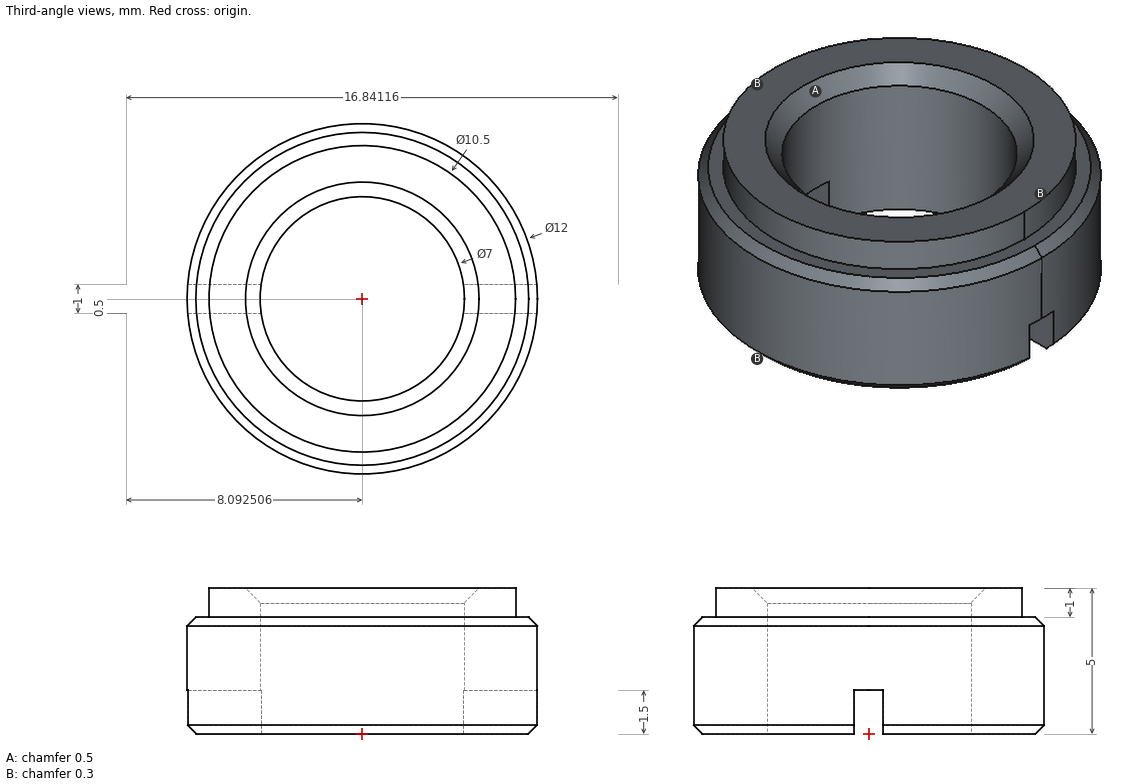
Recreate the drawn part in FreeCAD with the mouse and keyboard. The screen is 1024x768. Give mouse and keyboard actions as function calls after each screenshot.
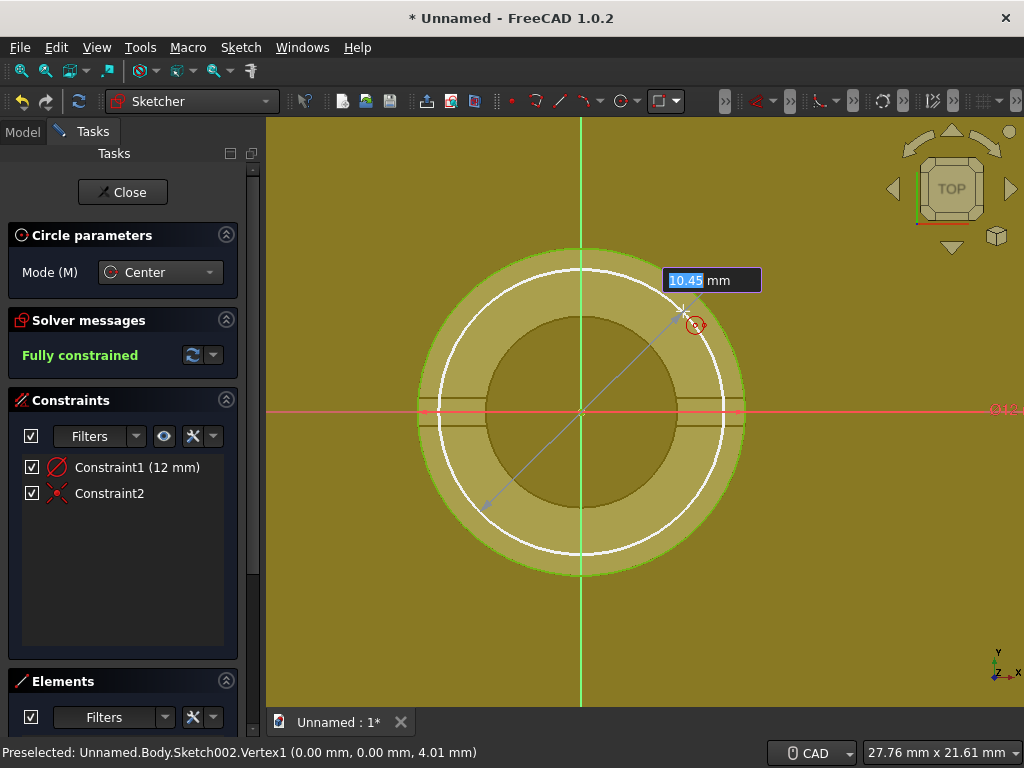
text(10.5)
key(Return)
key(Escape)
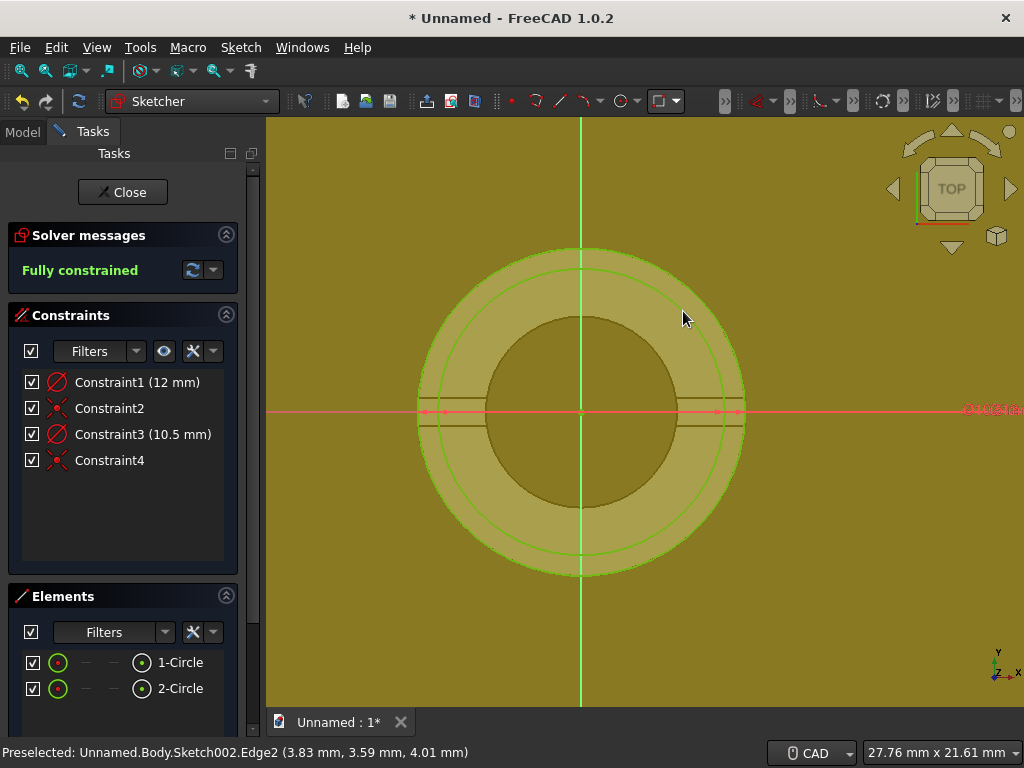
click(123, 192)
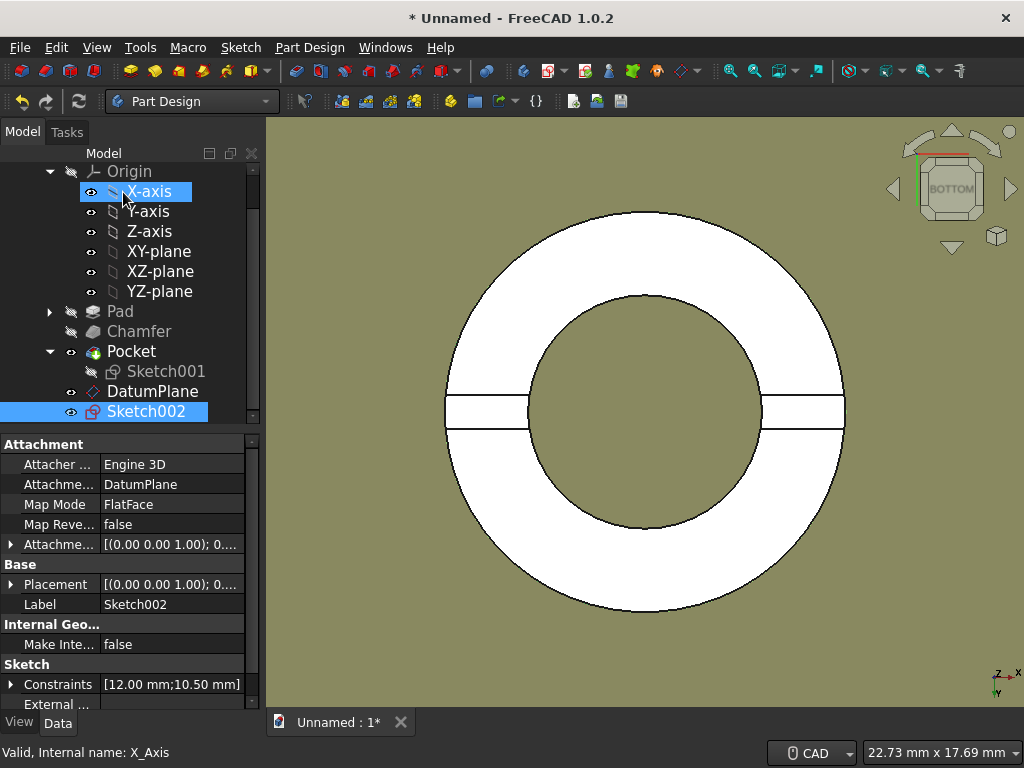
click(298, 72)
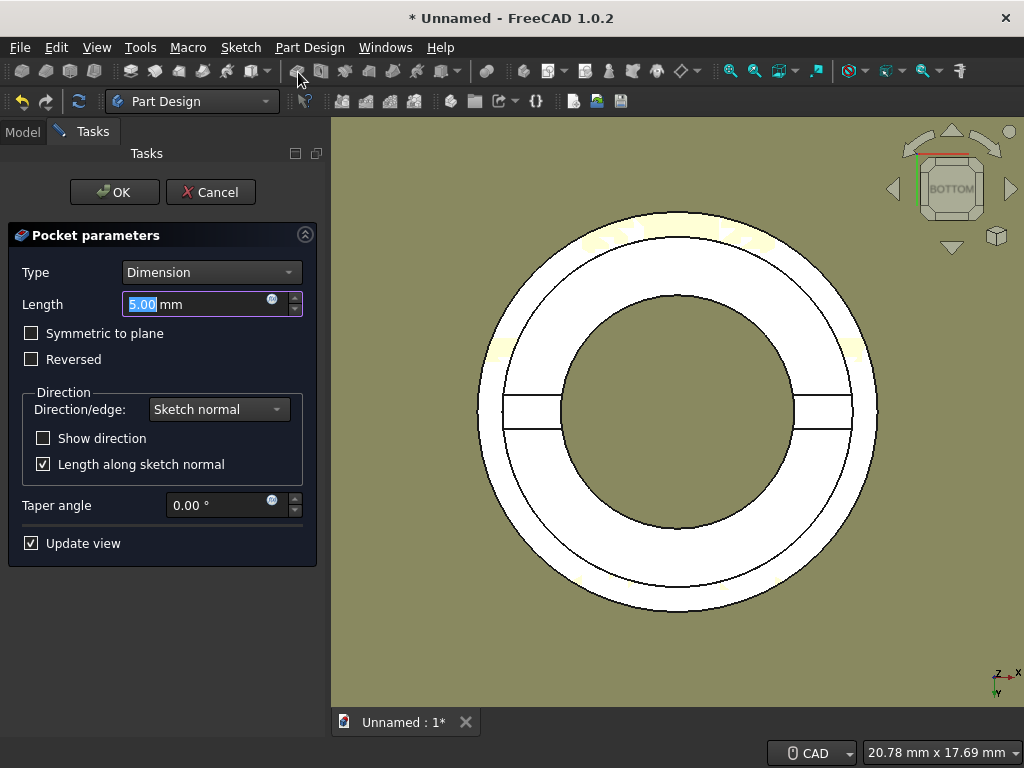
text(1)
key(Tab)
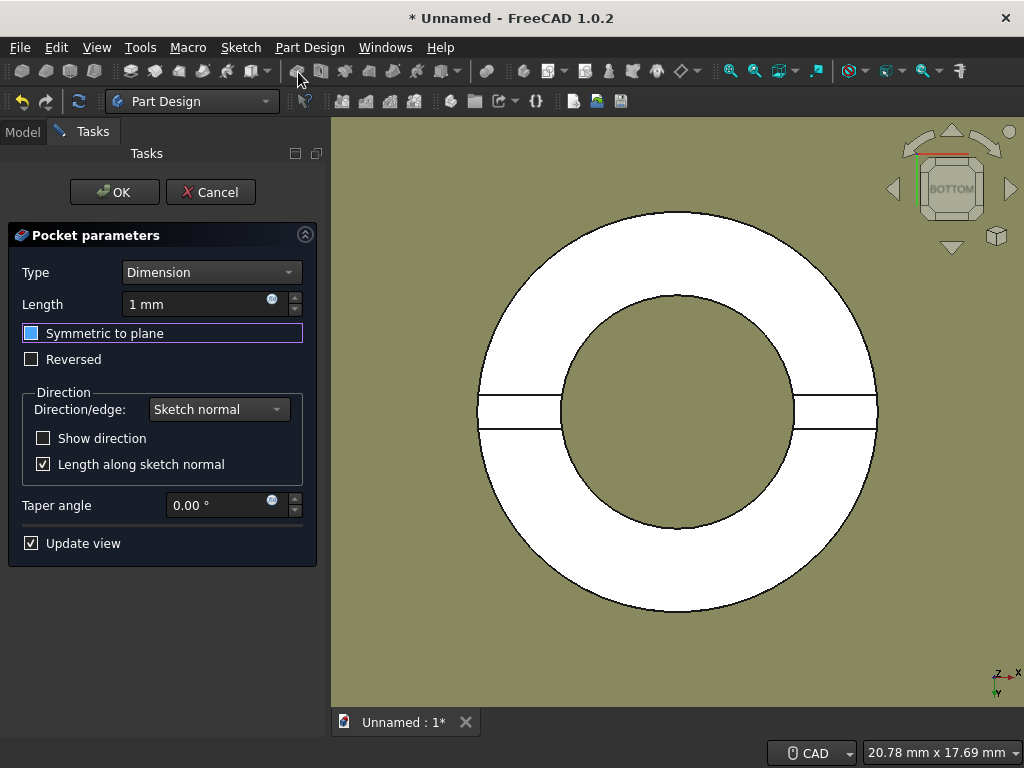
click(30, 359)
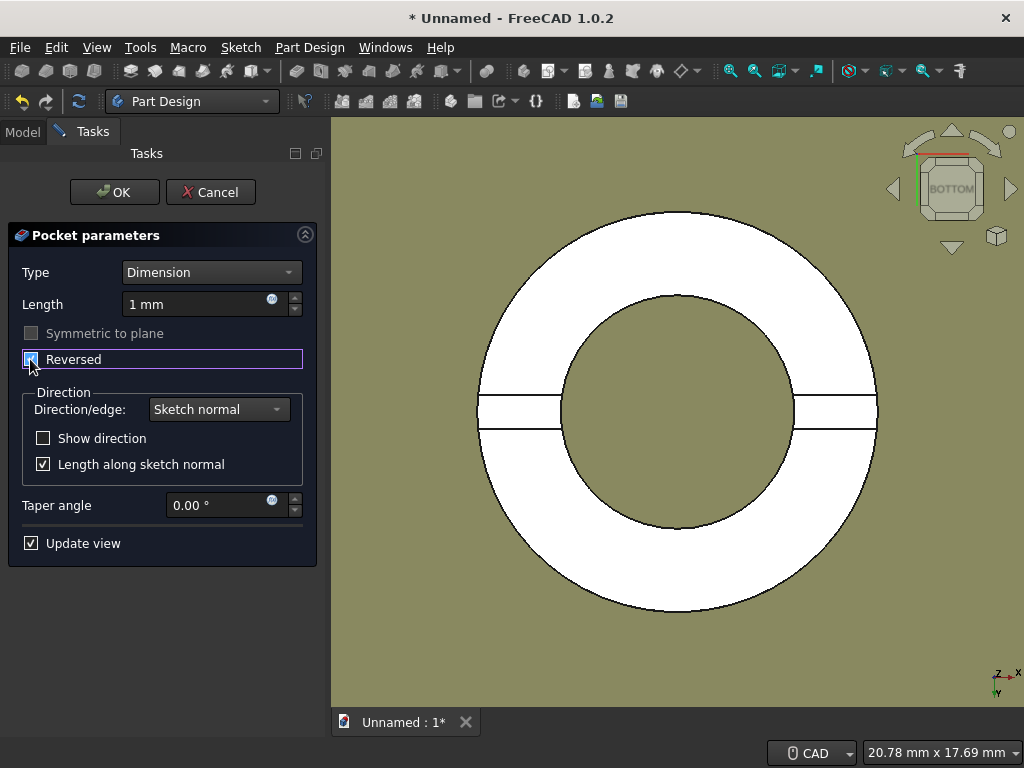
click(115, 192)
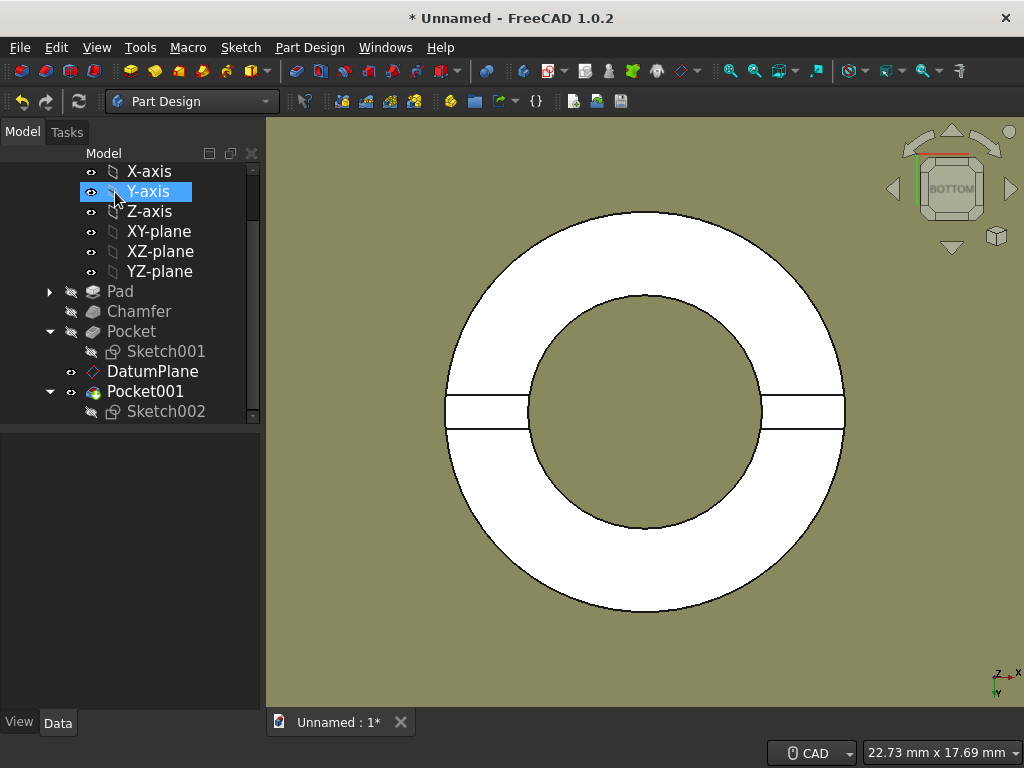
click(116, 372)
key(space)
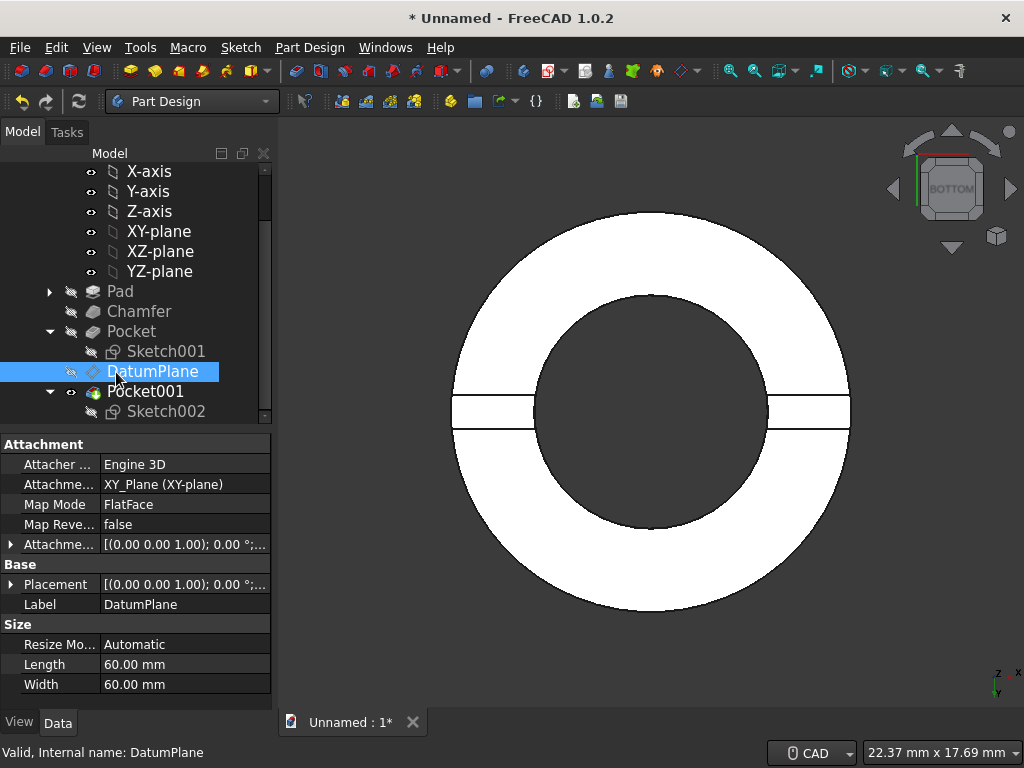
click(539, 245)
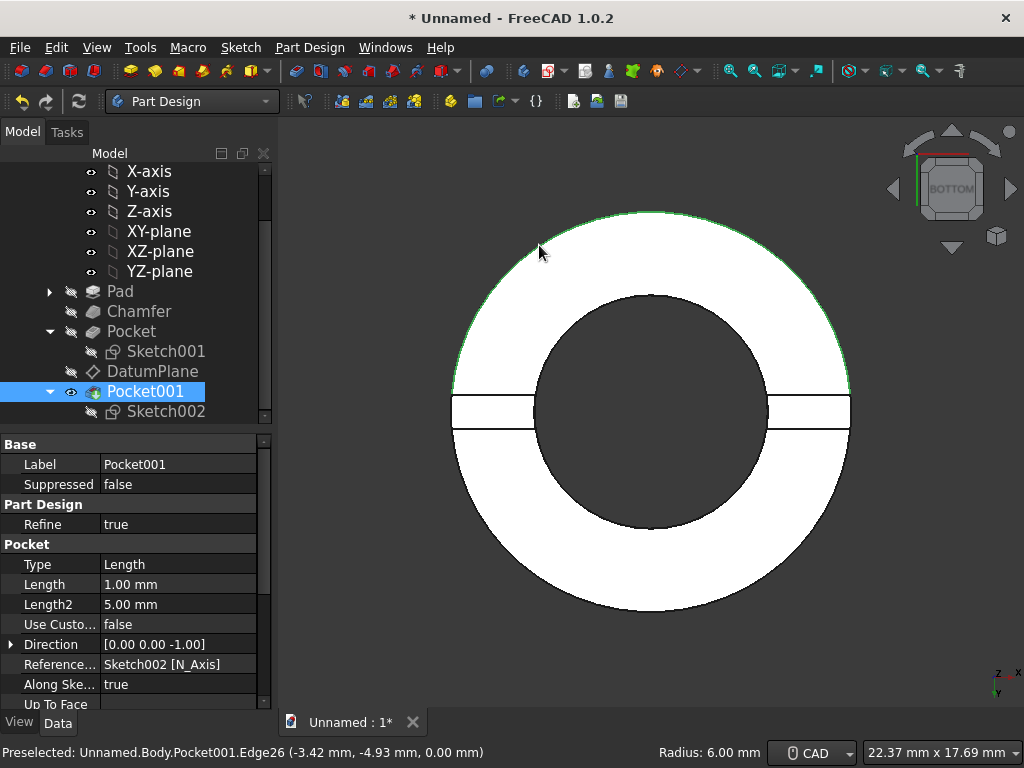
click(651, 611, ctrl)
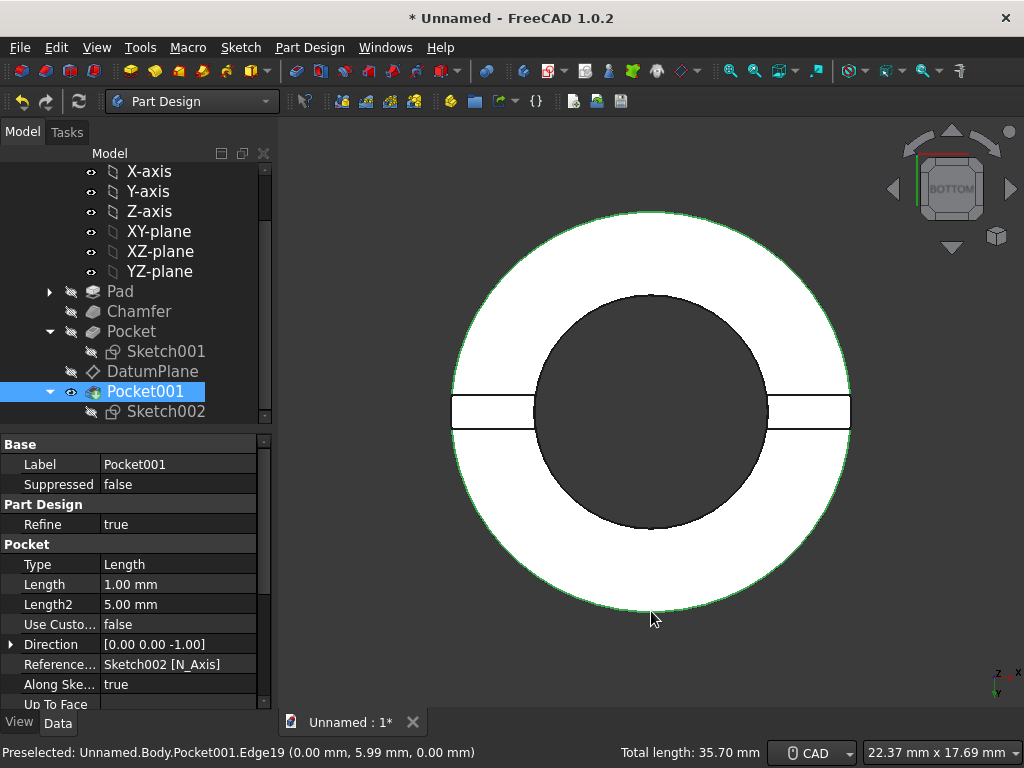
key(0)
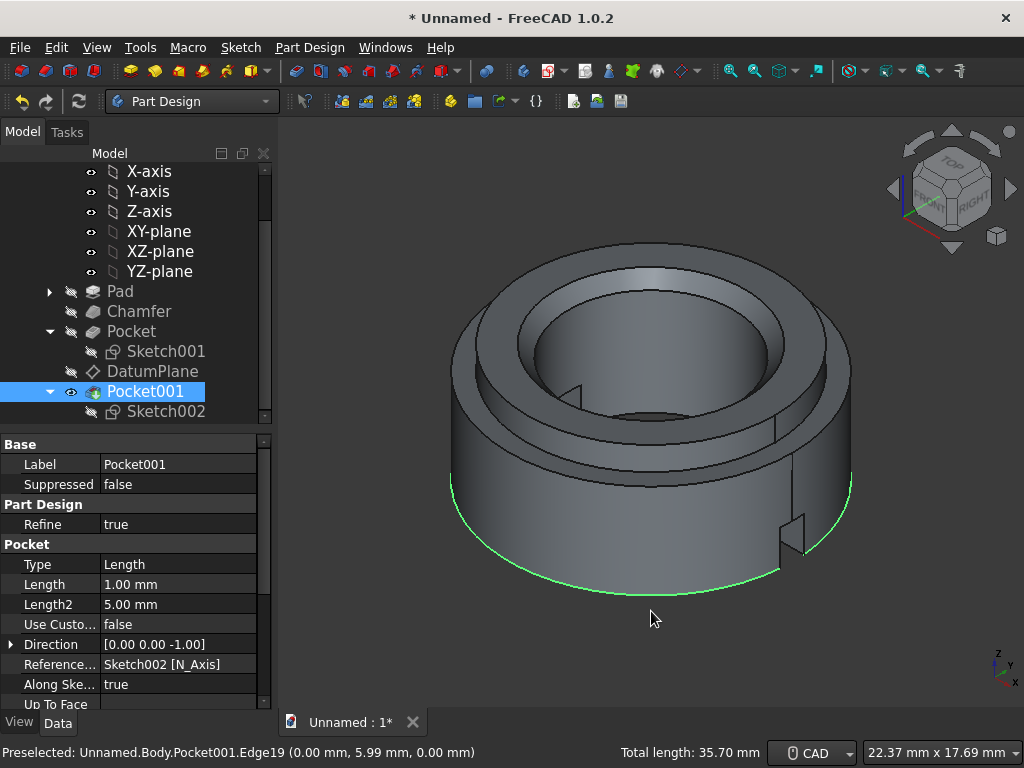
click(473, 423, ctrl)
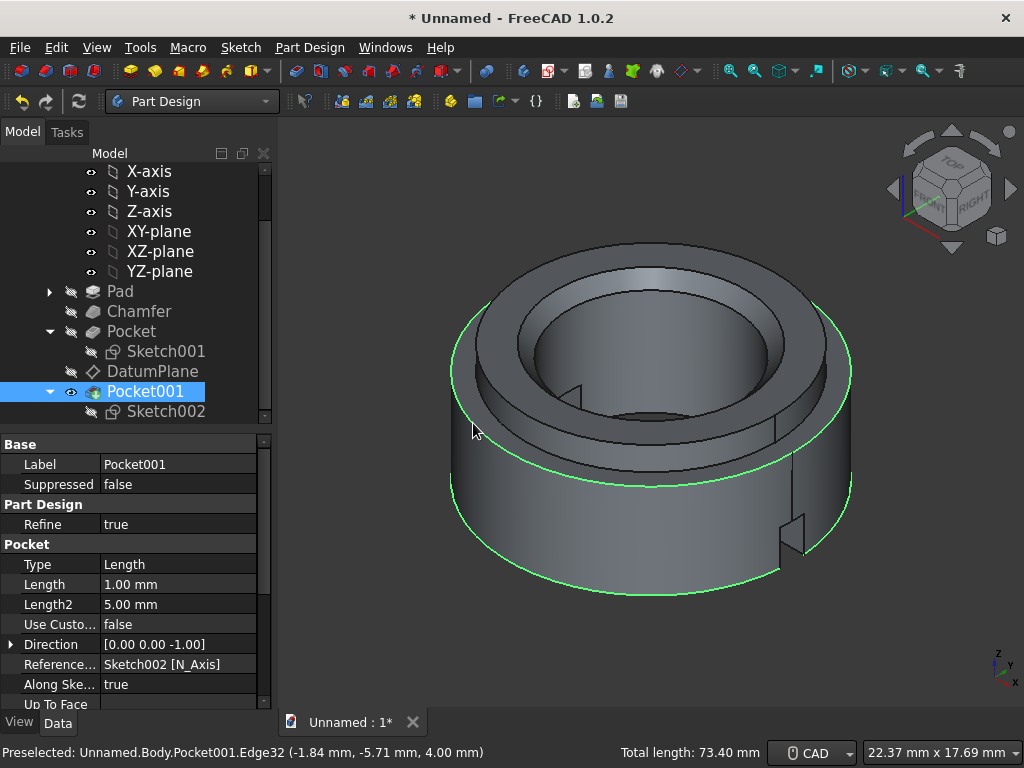
click(46, 72)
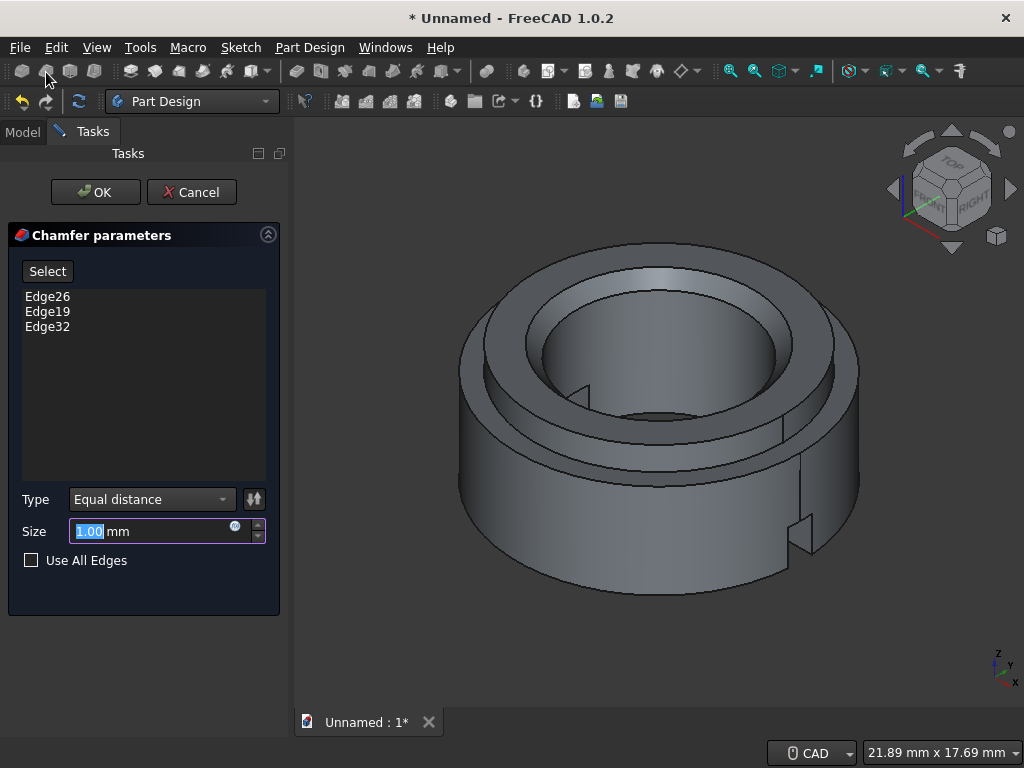
text(0.3)
key(Tab)